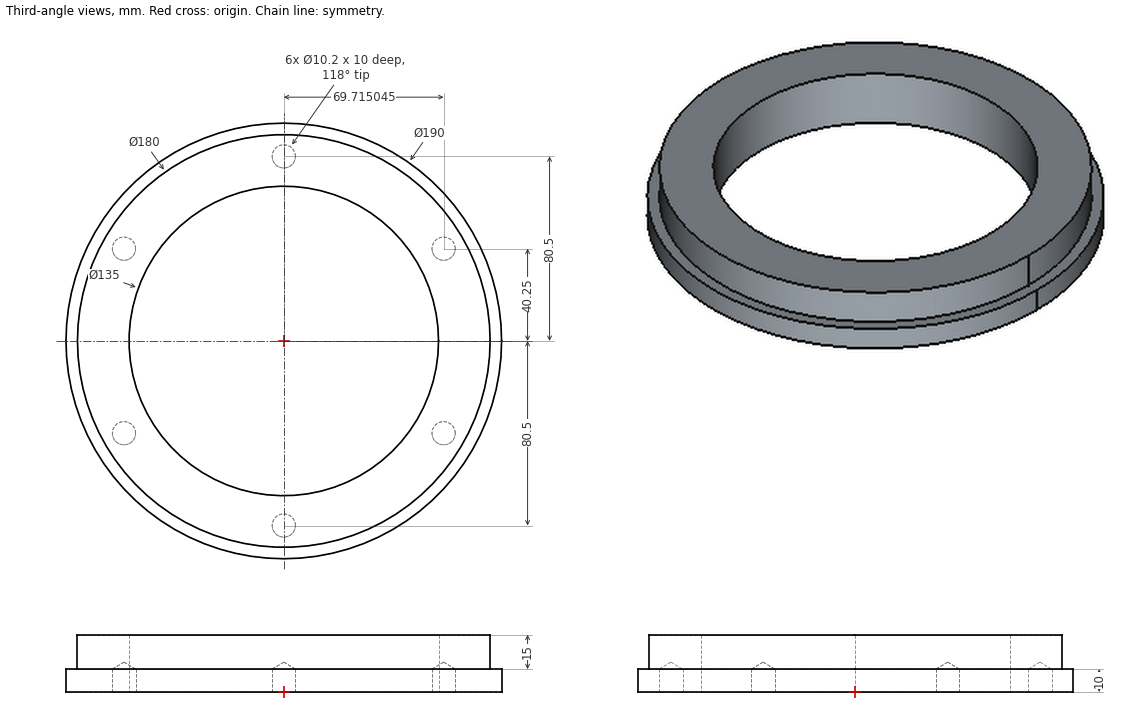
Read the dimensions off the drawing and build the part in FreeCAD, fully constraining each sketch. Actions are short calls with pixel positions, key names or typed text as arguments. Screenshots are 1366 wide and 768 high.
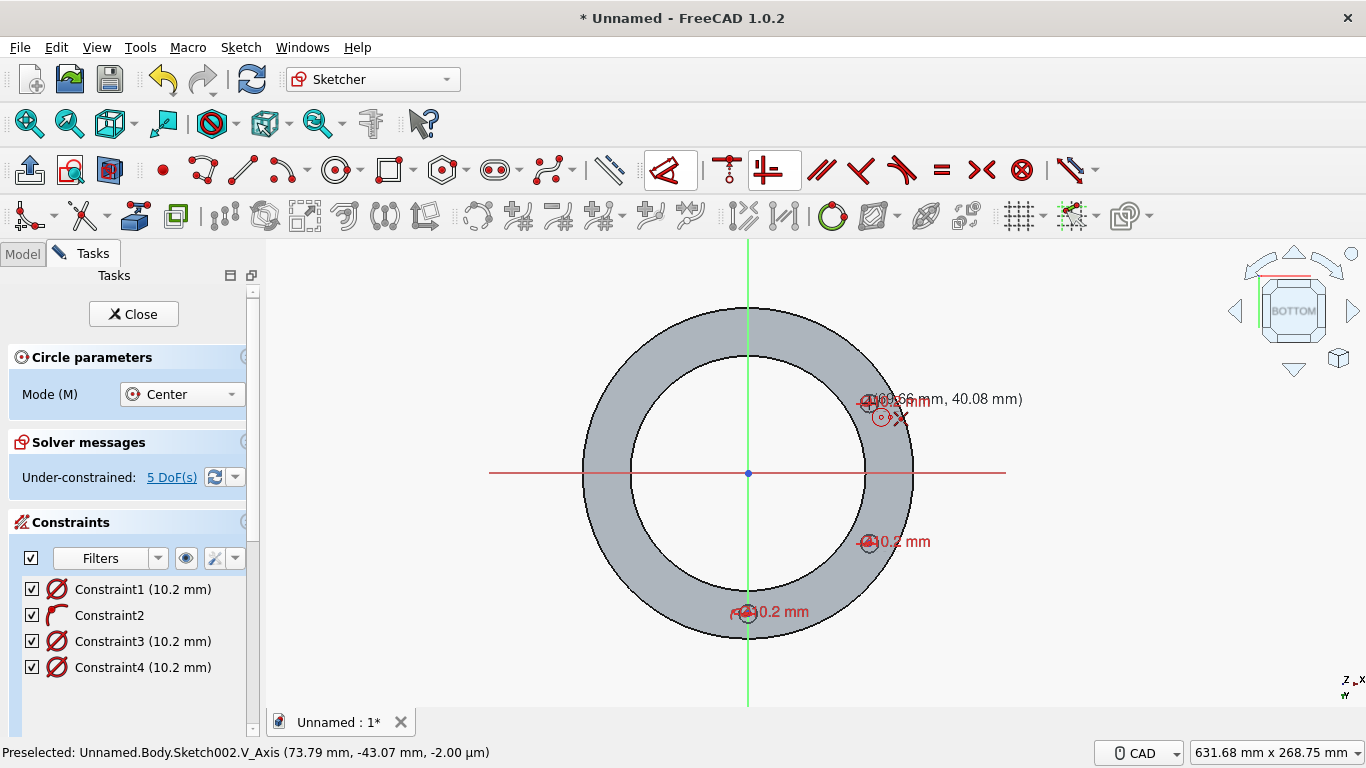
scroll(748, 333, up, 5)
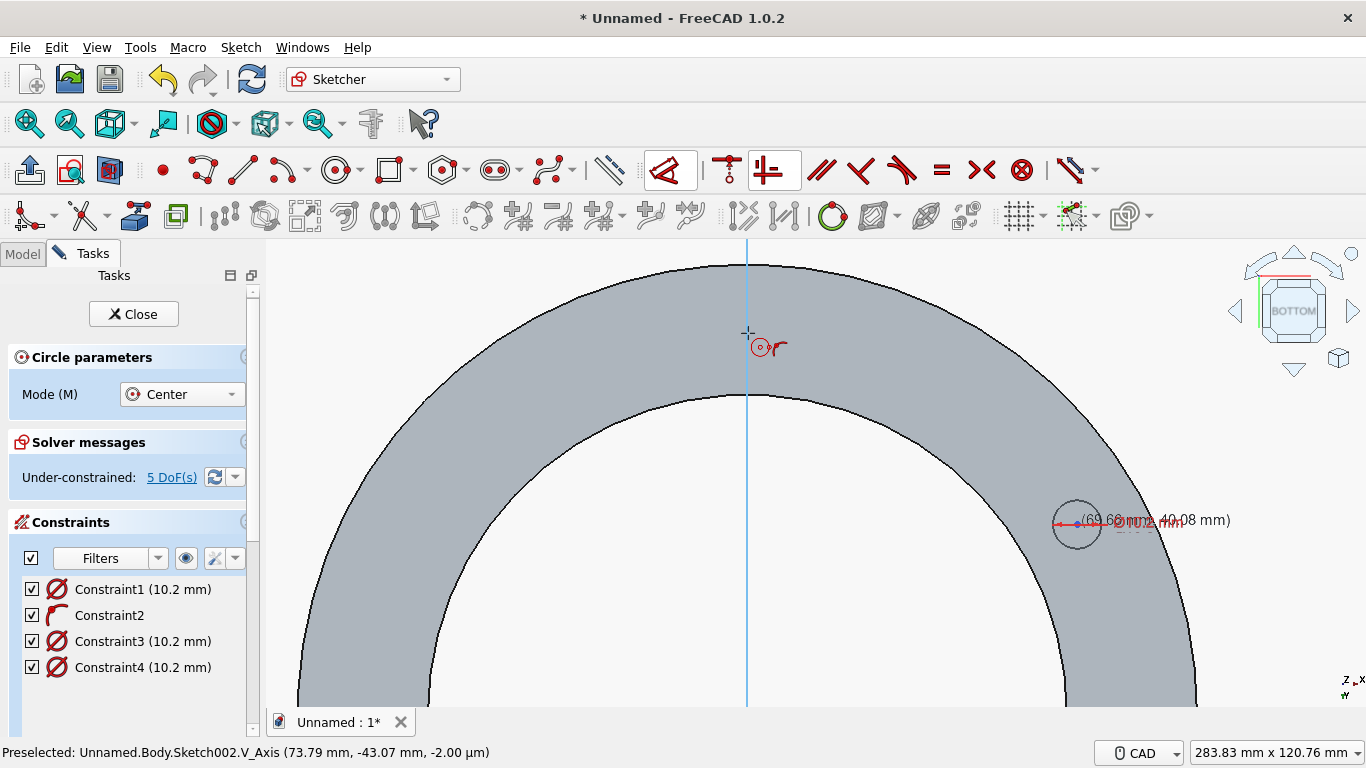
click(747, 333)
move(764, 316)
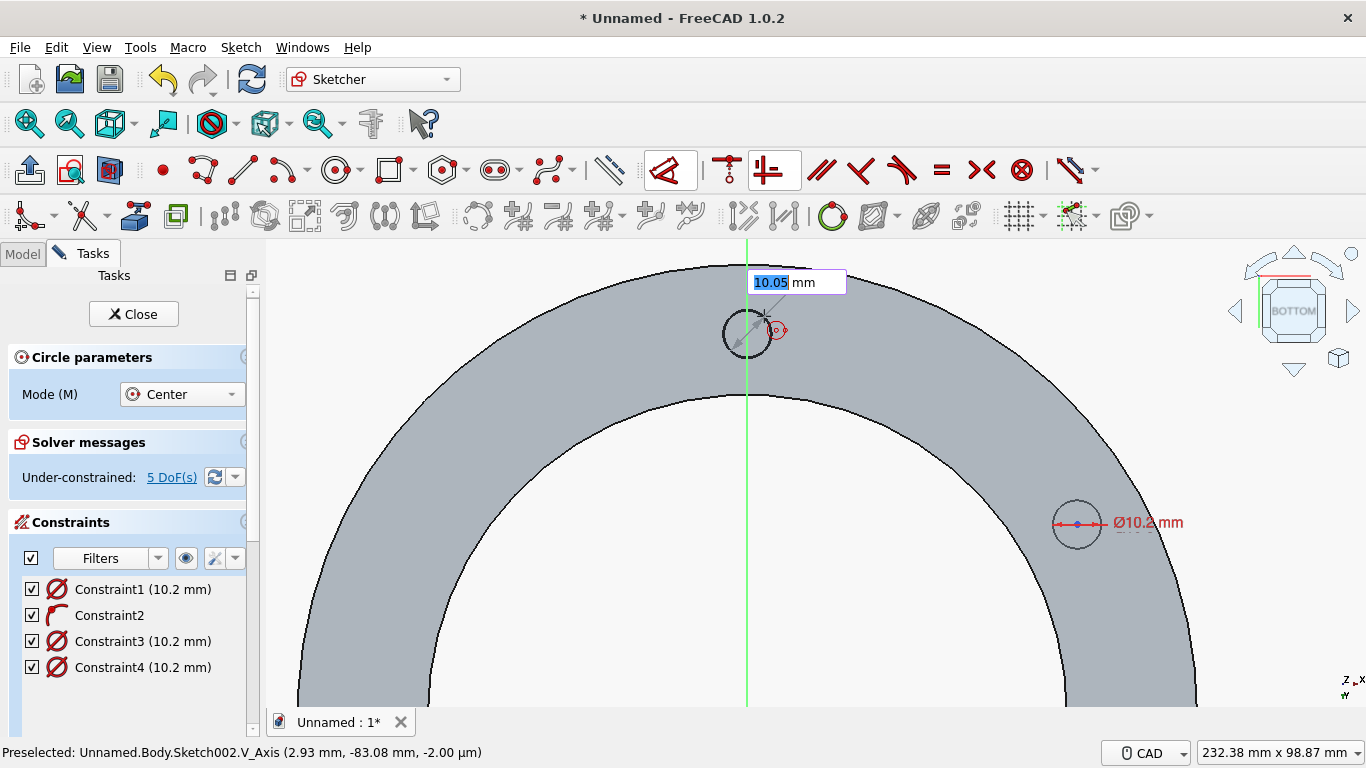
text(10.2)
key(Return)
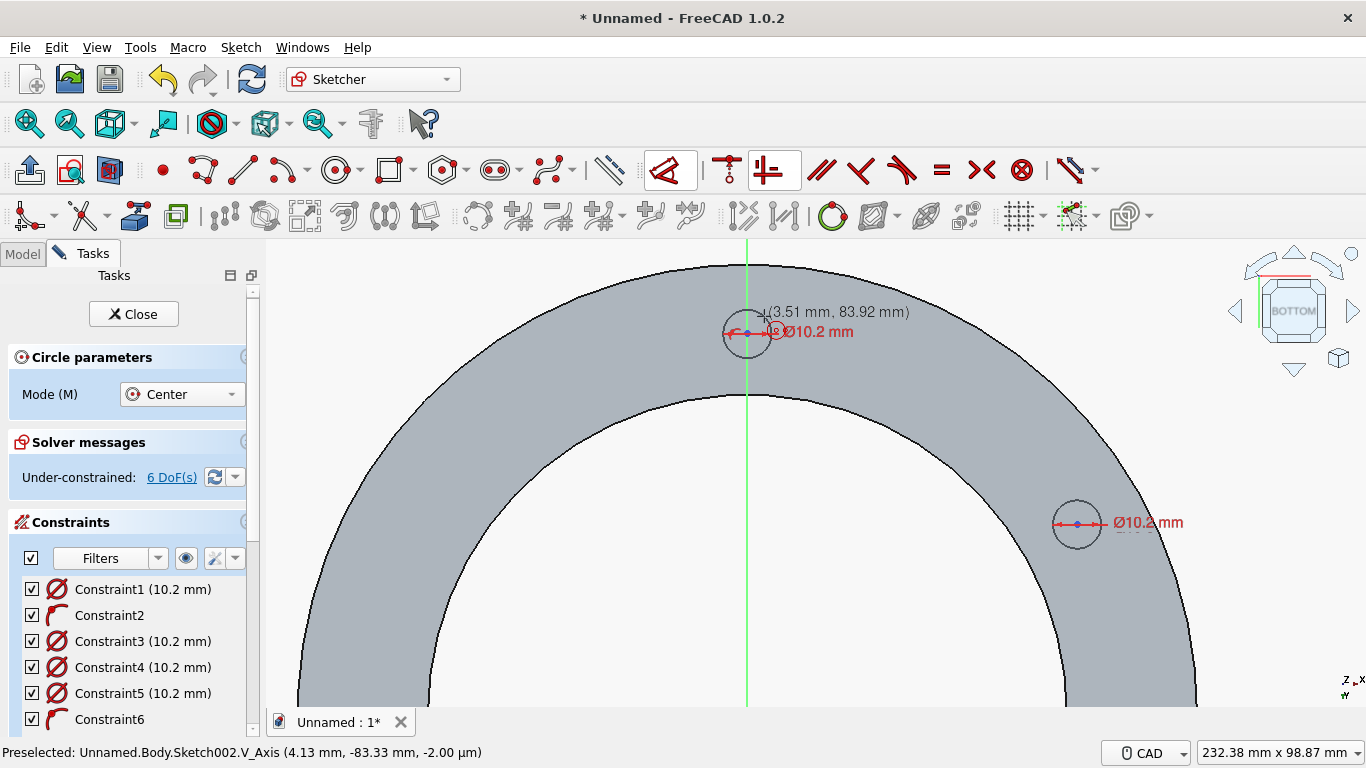
click(417, 524)
move(434, 507)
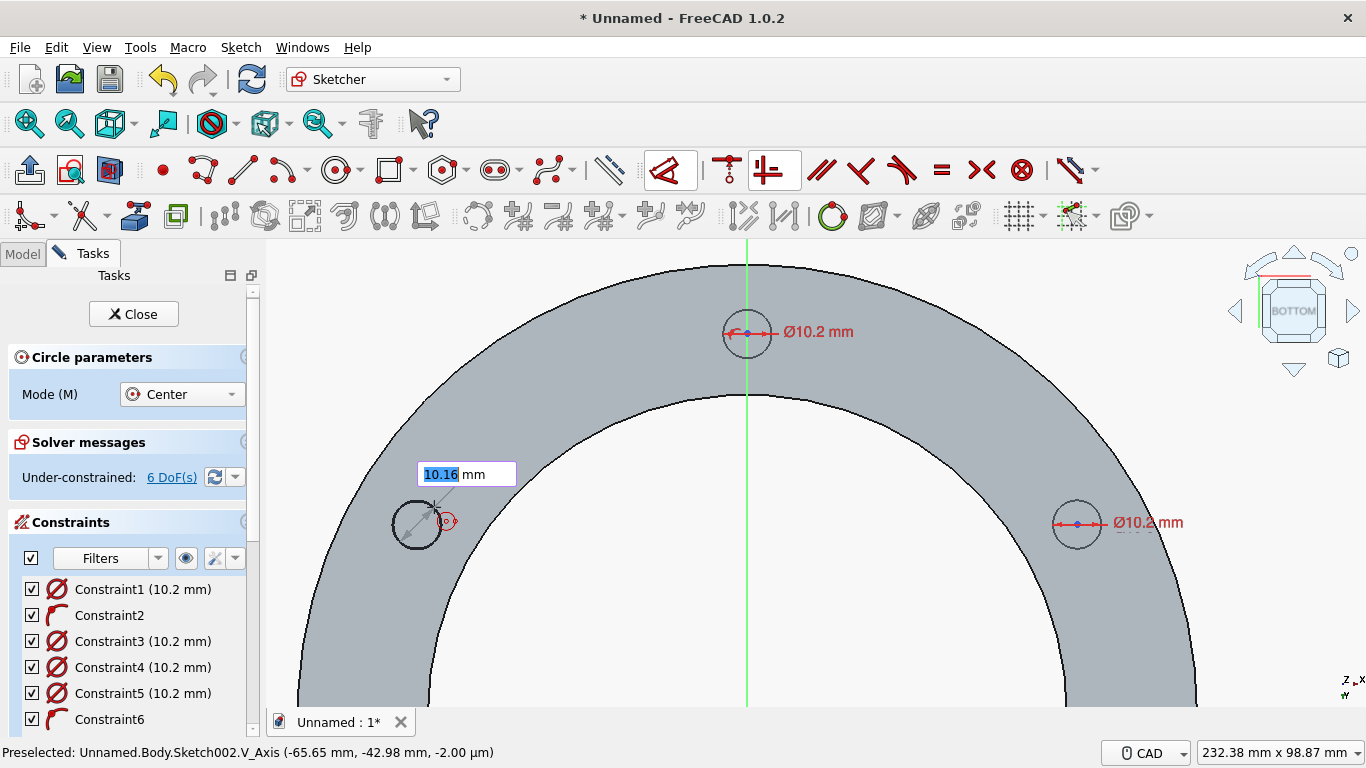
text(10.2)
key(Return)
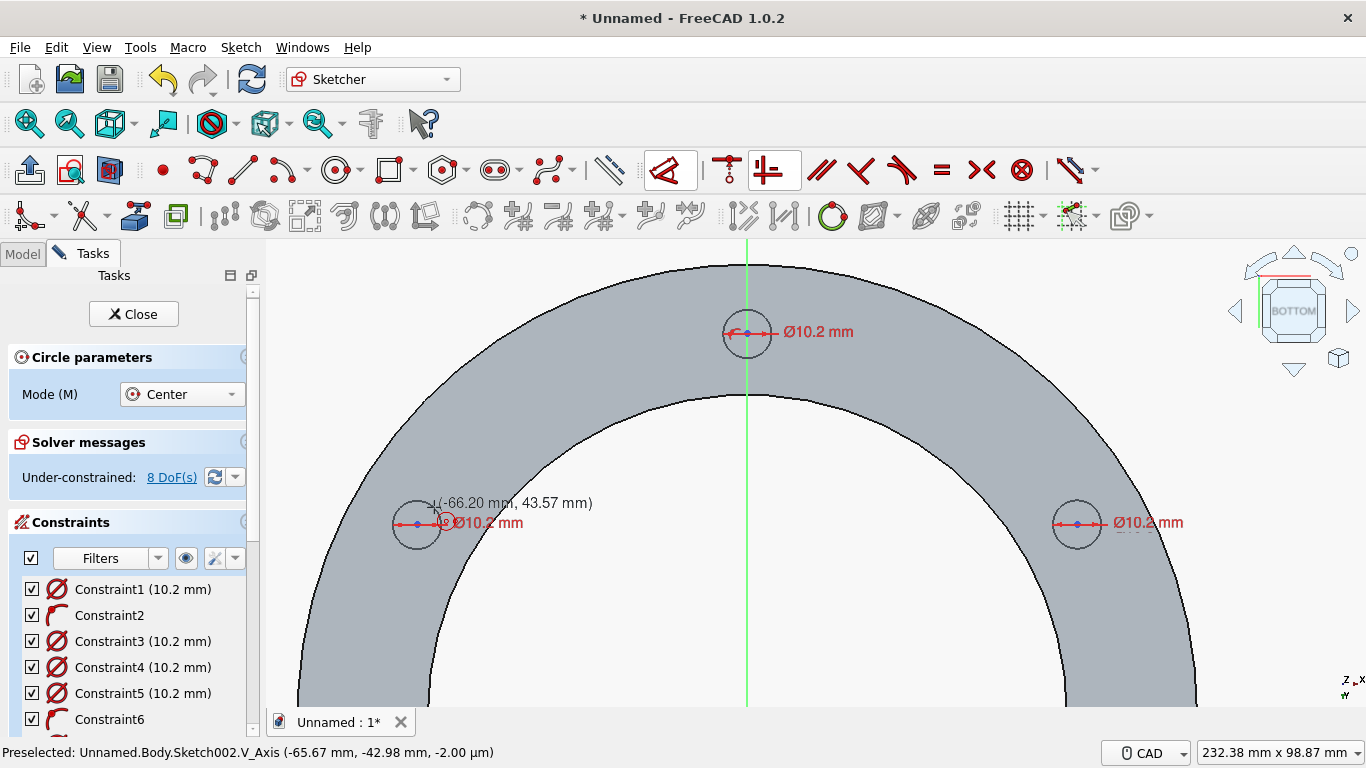
scroll(748, 333, down, 5)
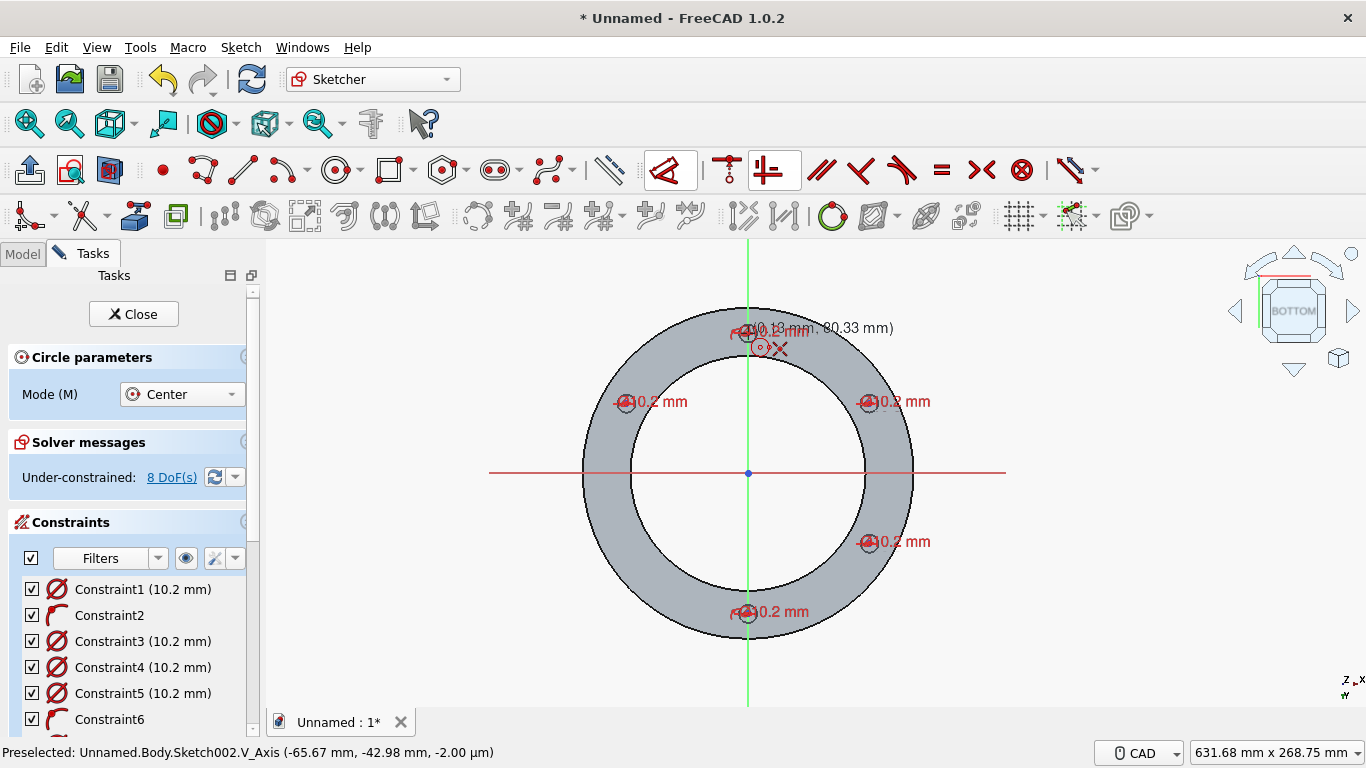
scroll(627, 543, up, 5)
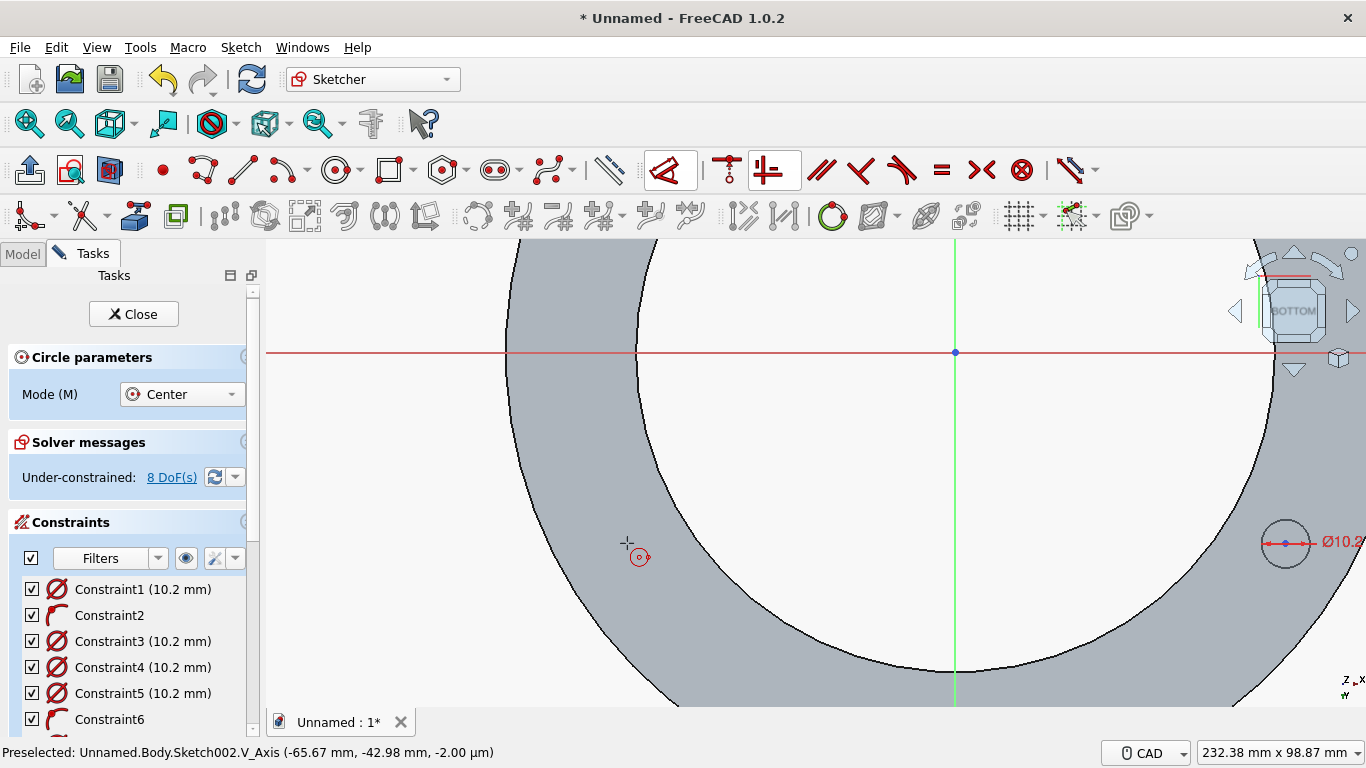
click(625, 543)
move(643, 526)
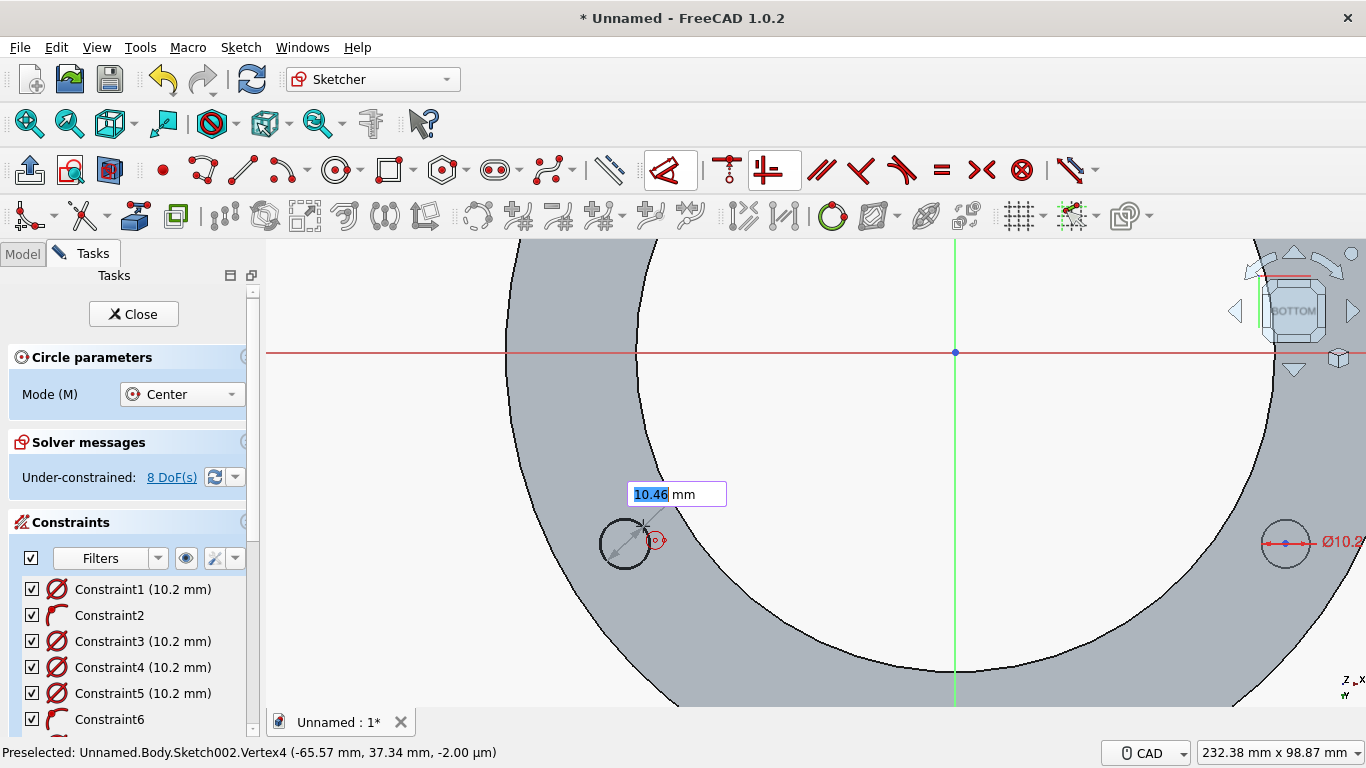
text(10.2)
key(Return)
key(Escape)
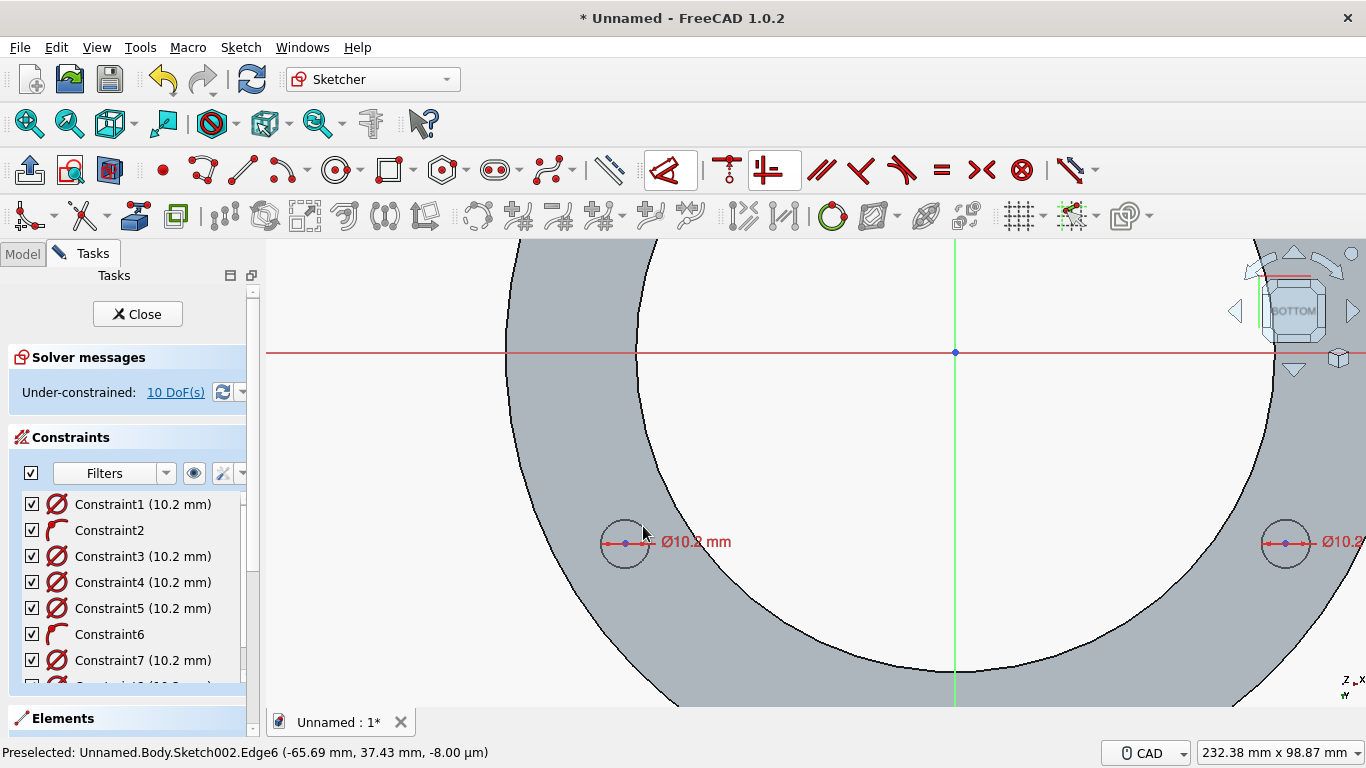
scroll(626, 543, down, 5)